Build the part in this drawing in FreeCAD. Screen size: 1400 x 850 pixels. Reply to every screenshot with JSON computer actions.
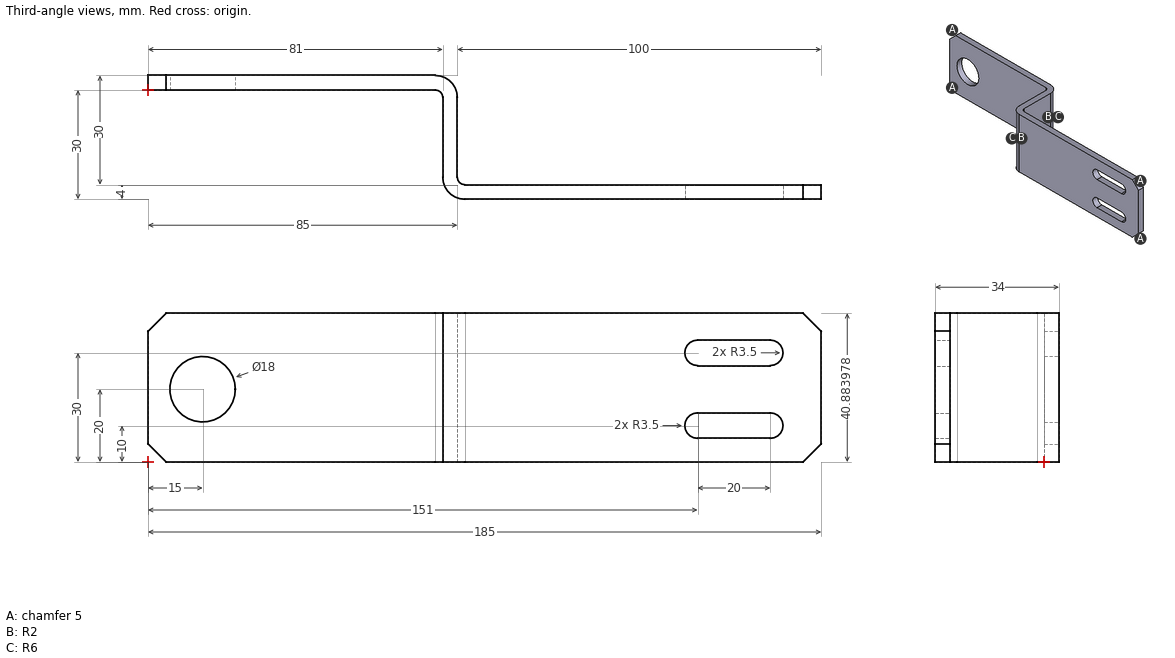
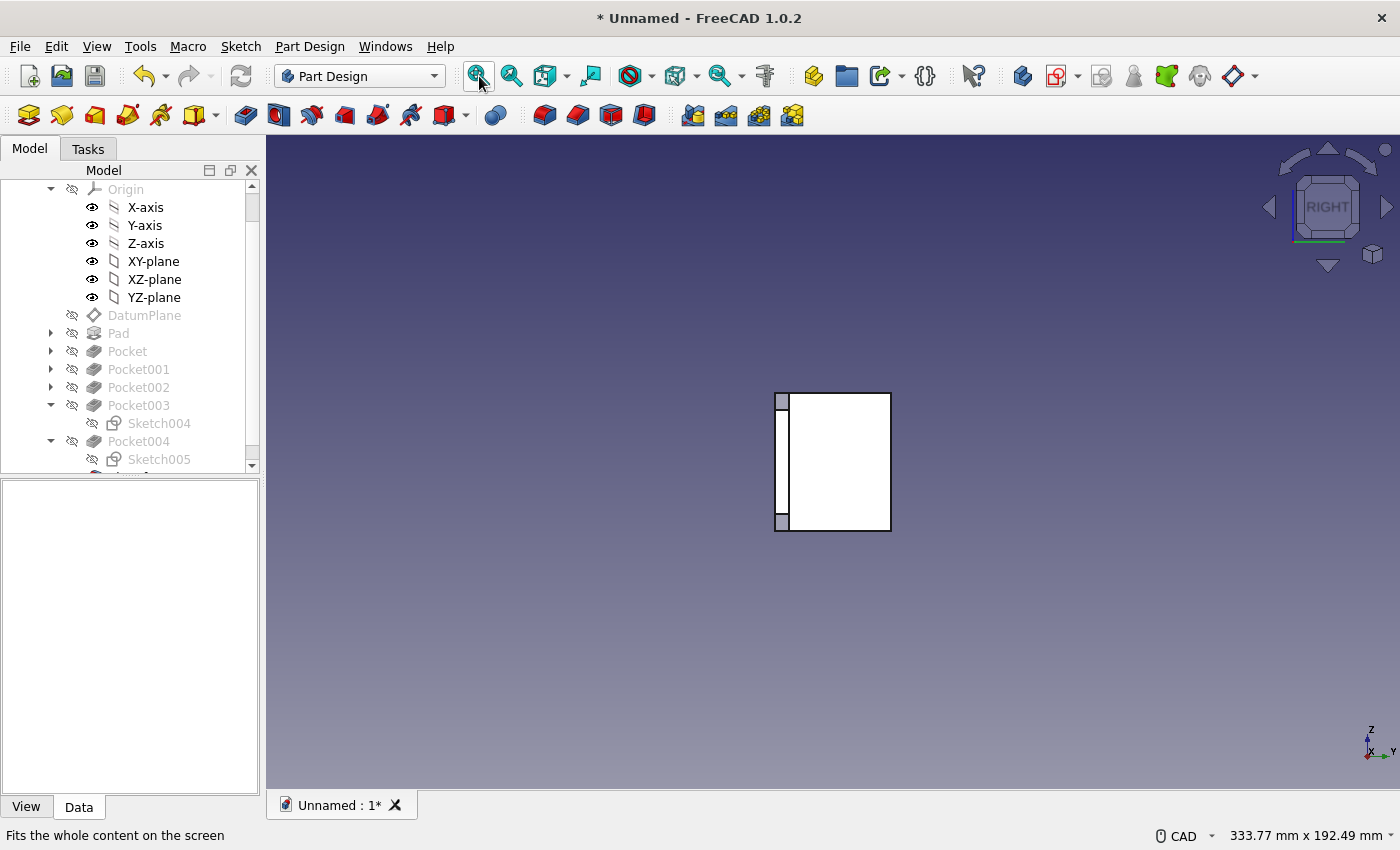
{"action": "key", "text": "5"}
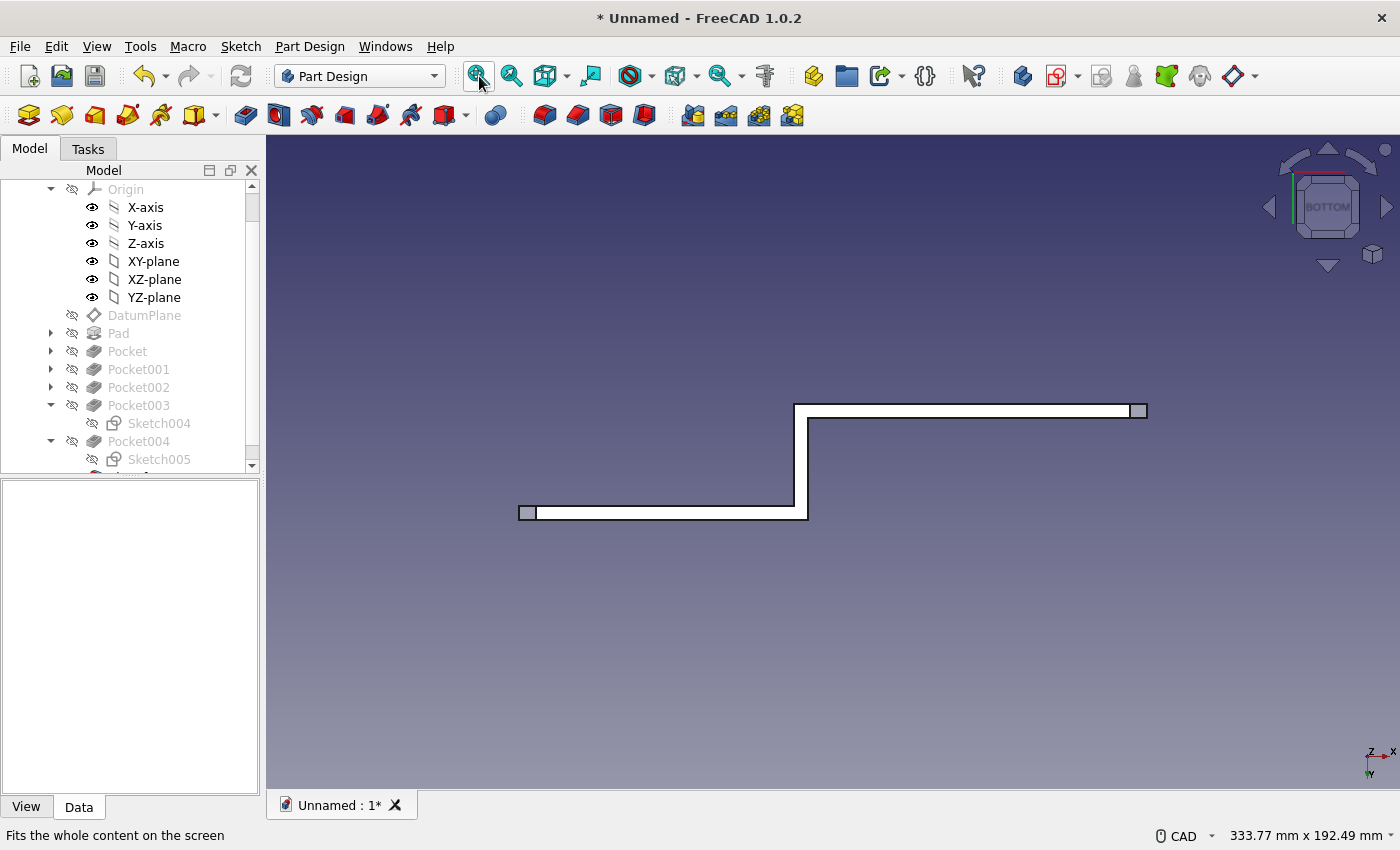
{"action": "key", "text": "4"}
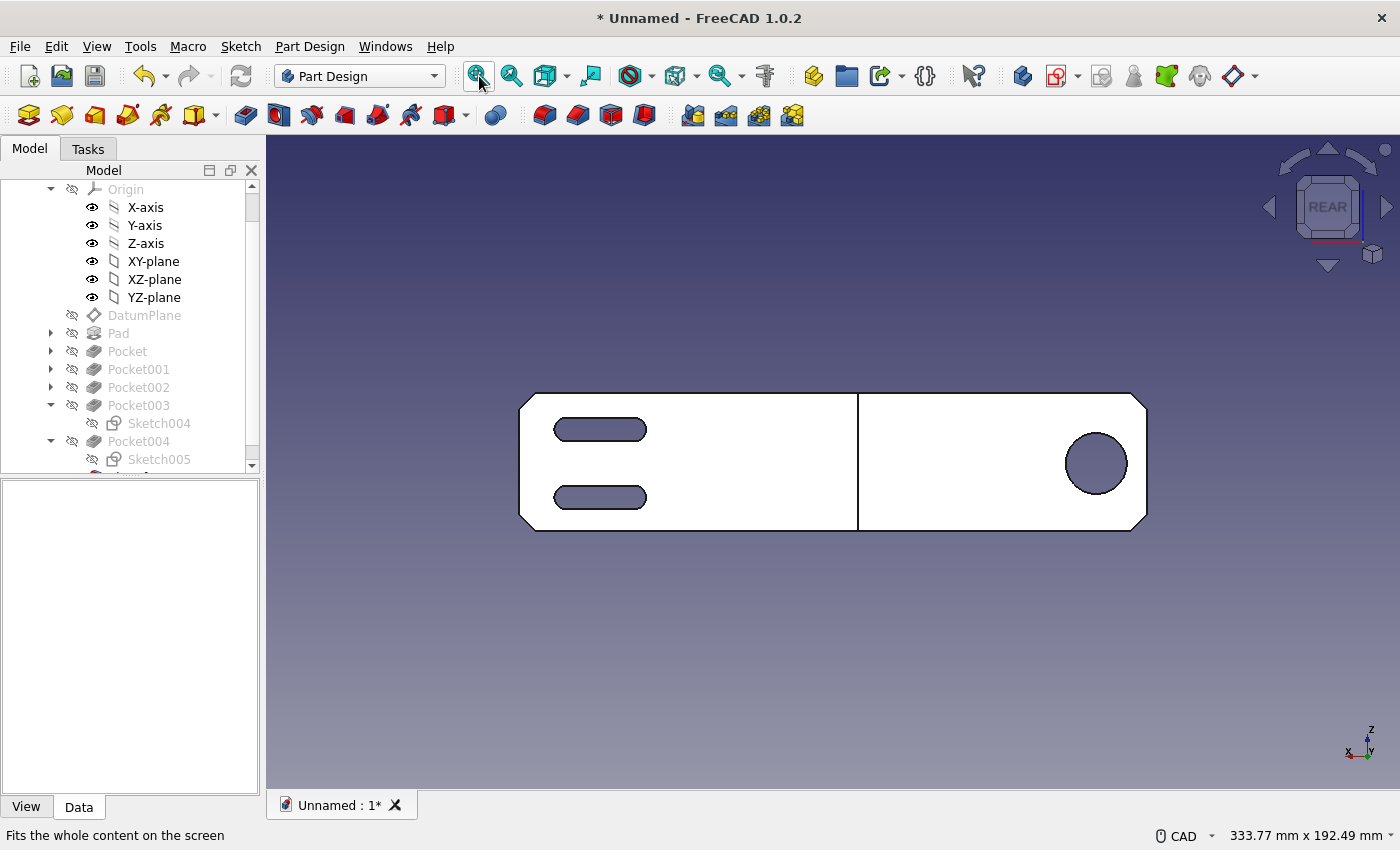
{"action": "key", "text": "6"}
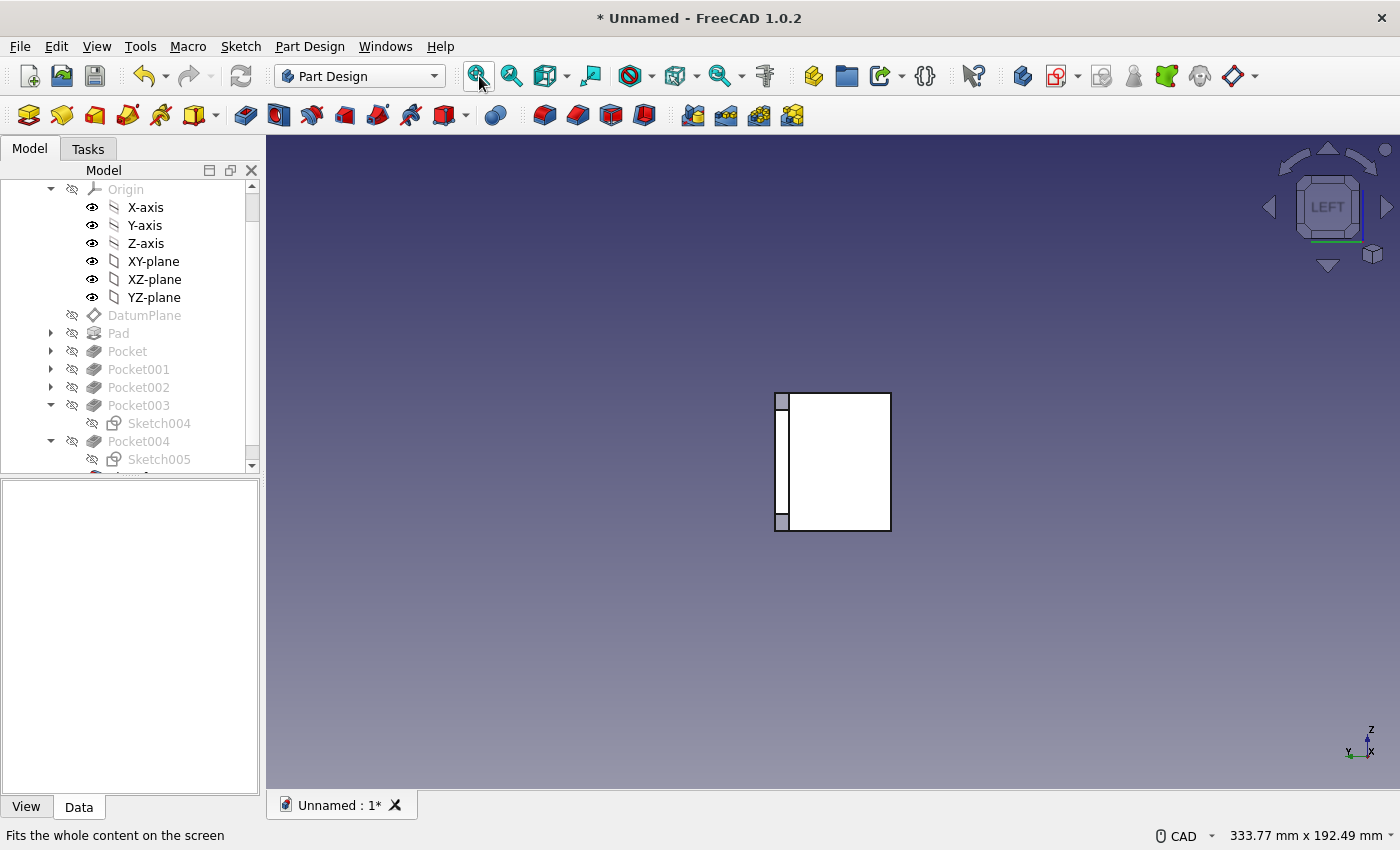
{"action": "key", "text": "v f"}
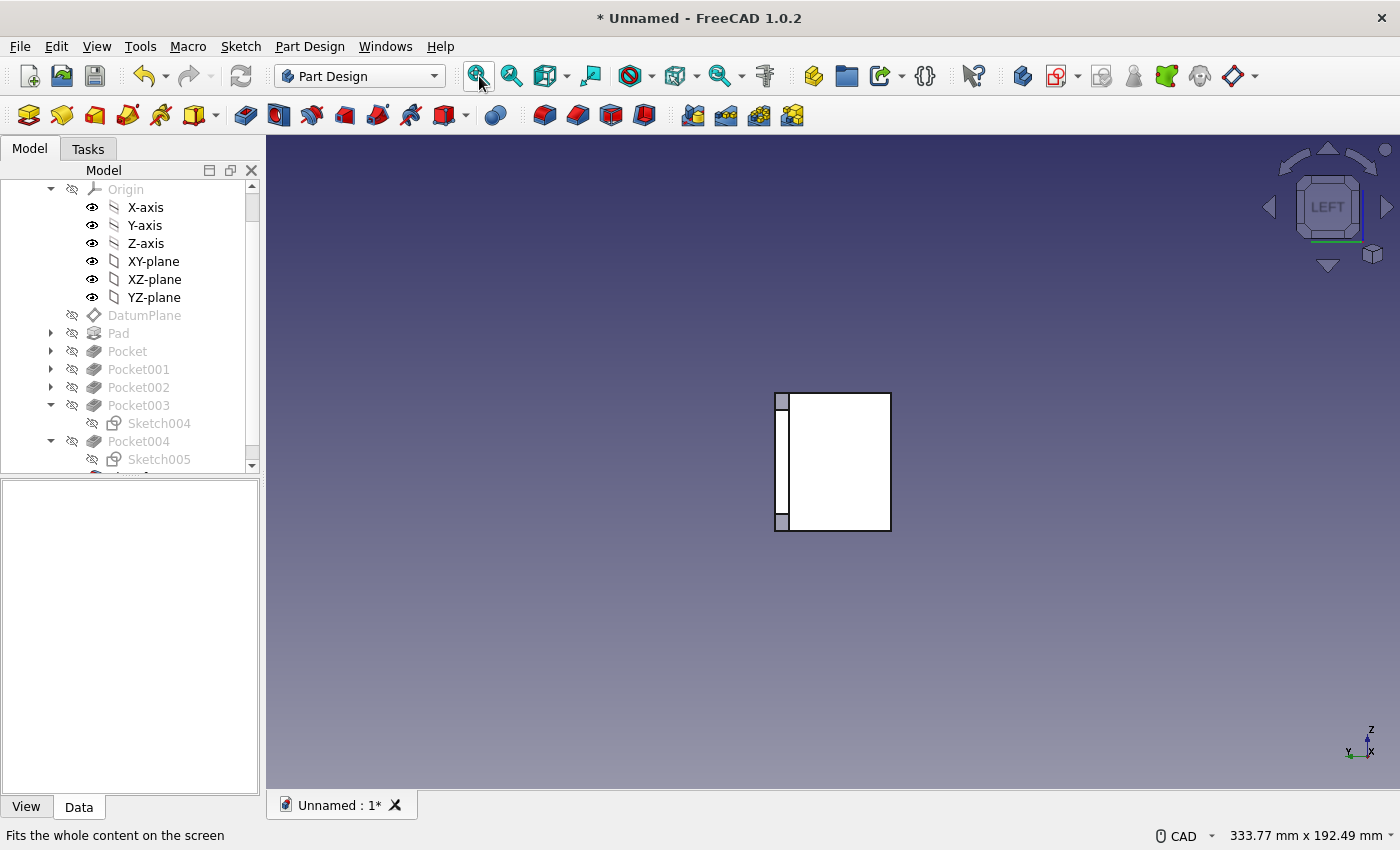
{"action": "key", "text": "v 3"}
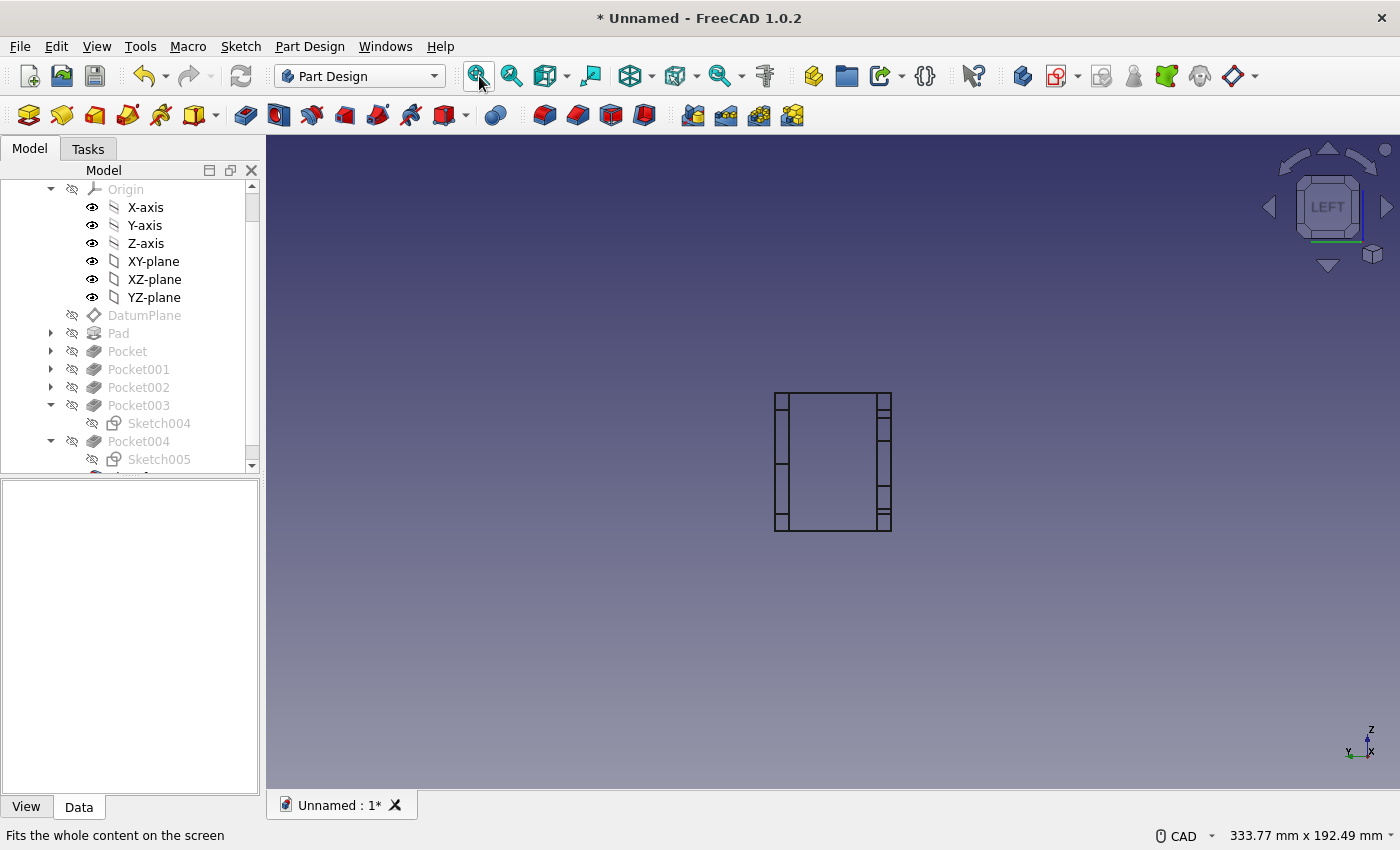
{"action": "key", "text": "0"}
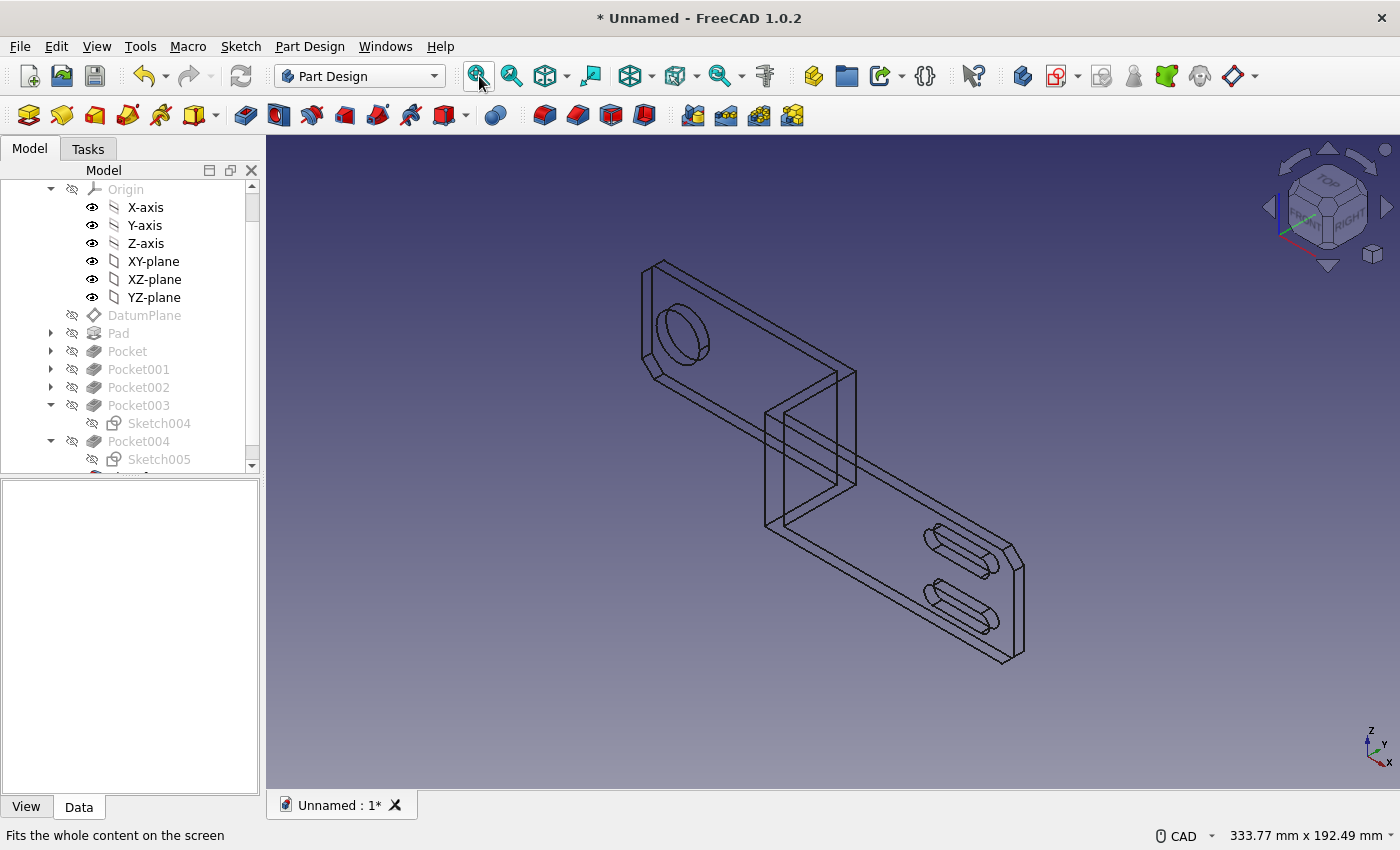
{"action": "left_click", "coordinate": [784, 469]}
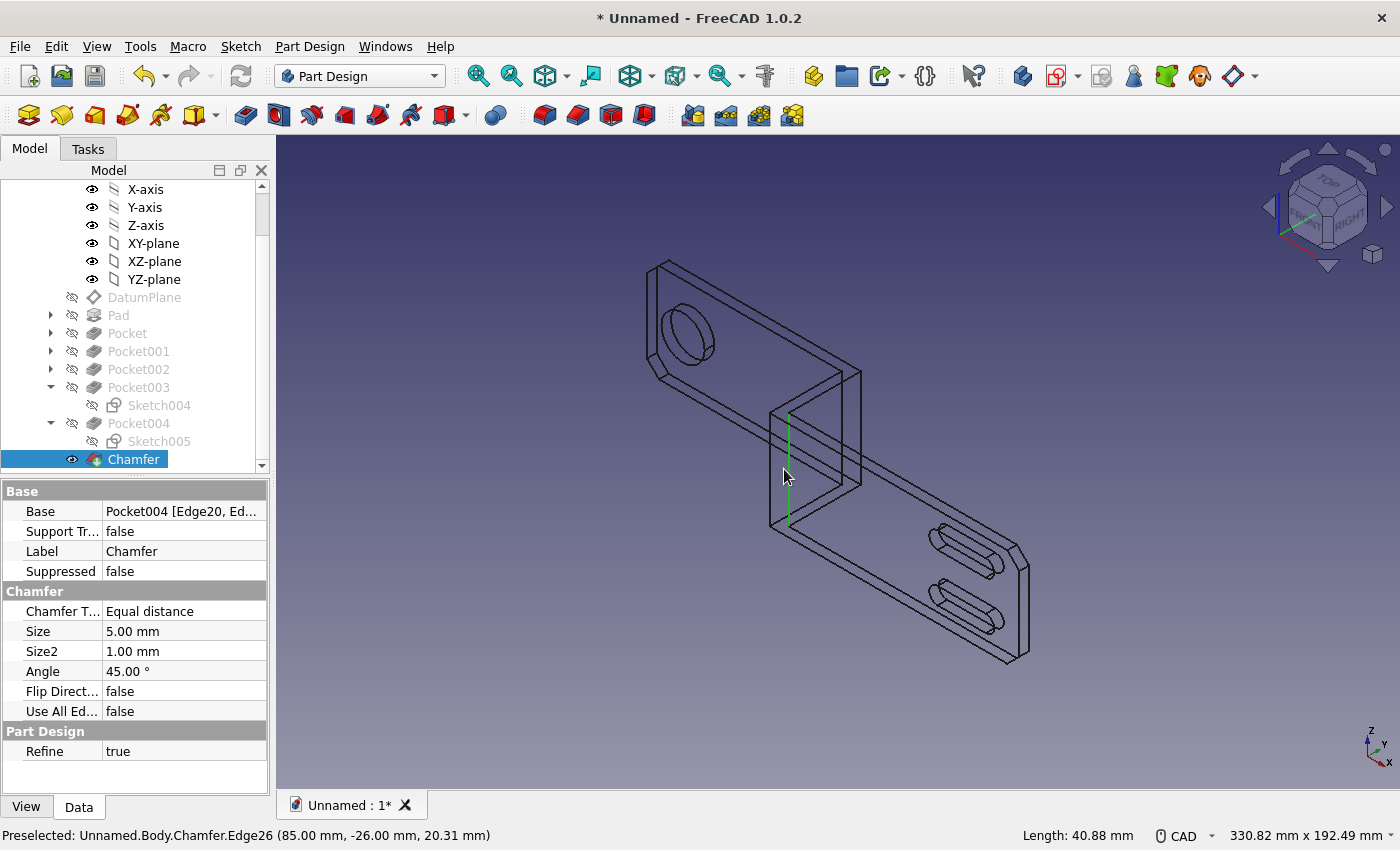
{"action": "left_click", "coordinate": [842, 427], "text": "ctrl"}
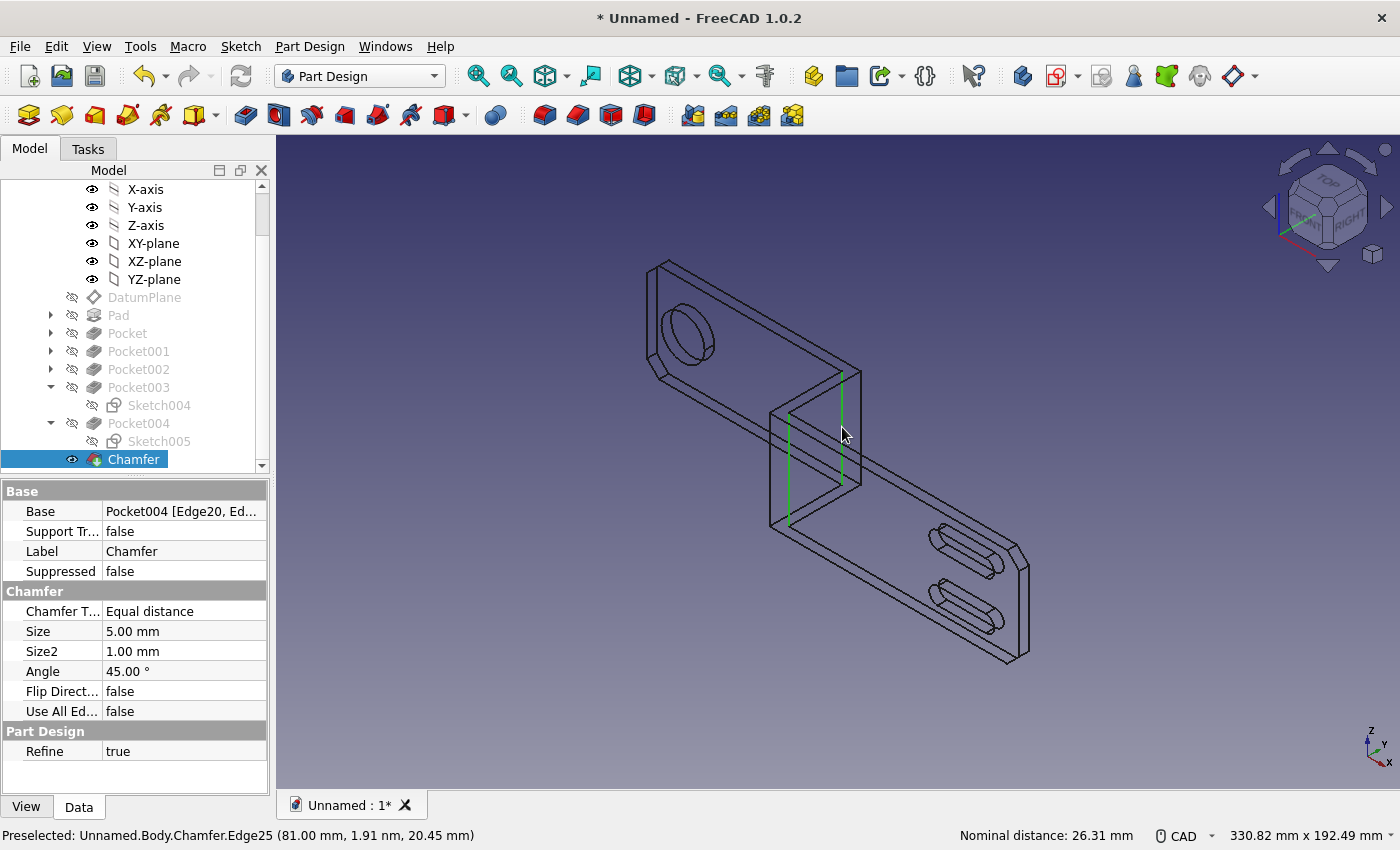
{"action": "key", "text": "v 1"}